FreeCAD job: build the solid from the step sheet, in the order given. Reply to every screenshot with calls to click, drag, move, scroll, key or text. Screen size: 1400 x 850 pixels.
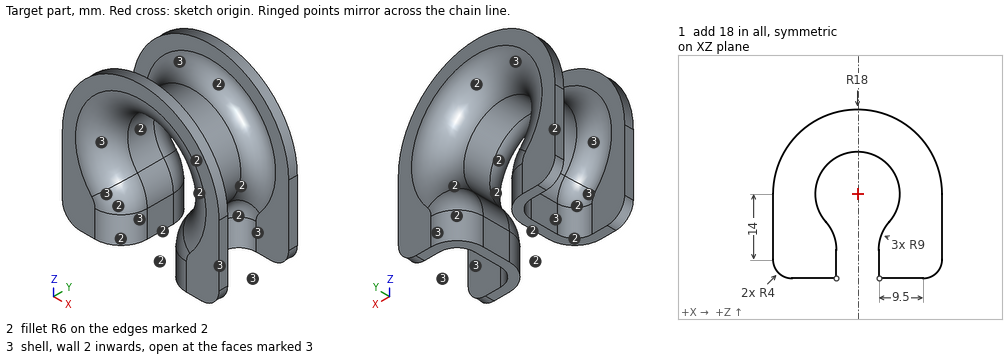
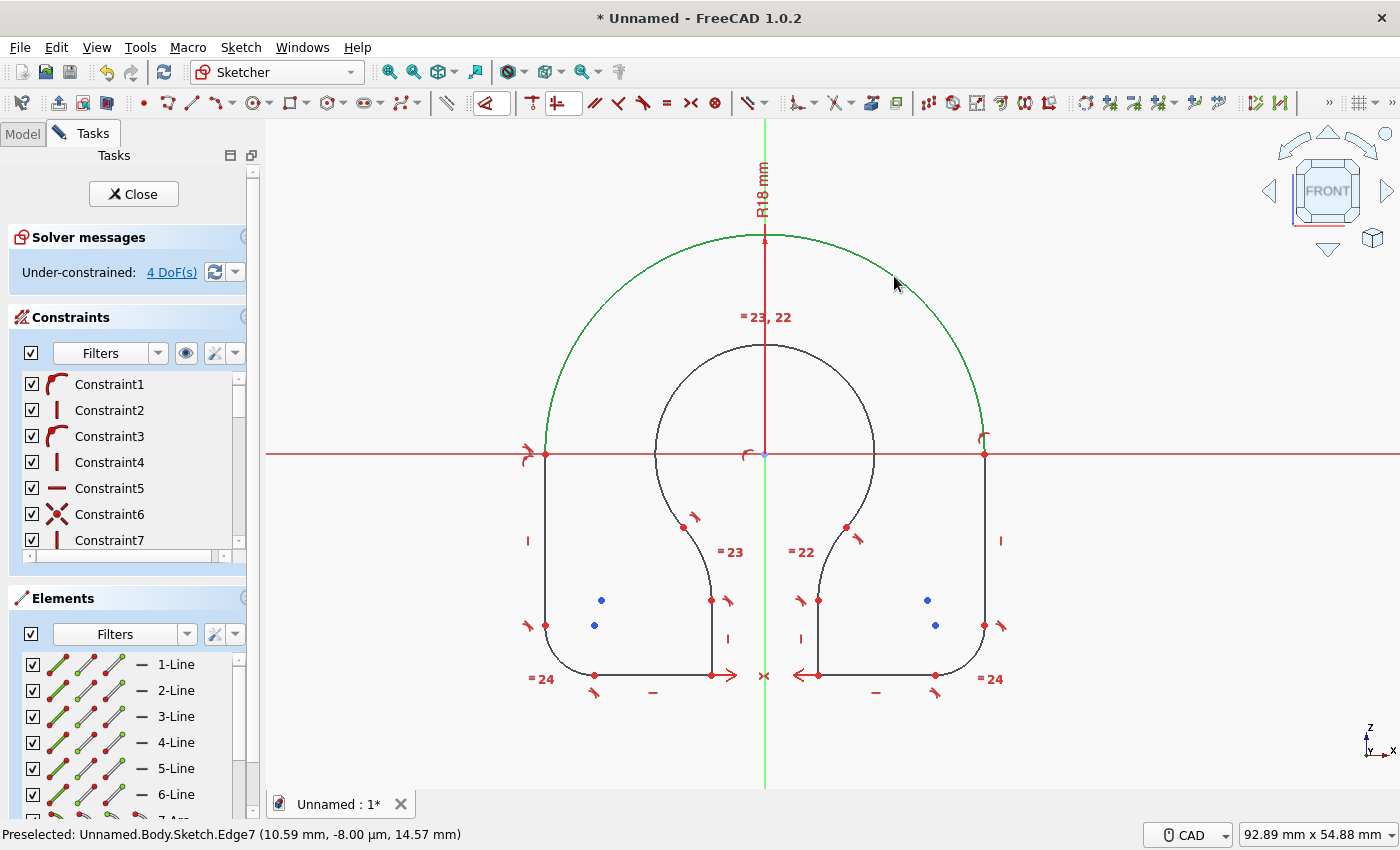
click(958, 670)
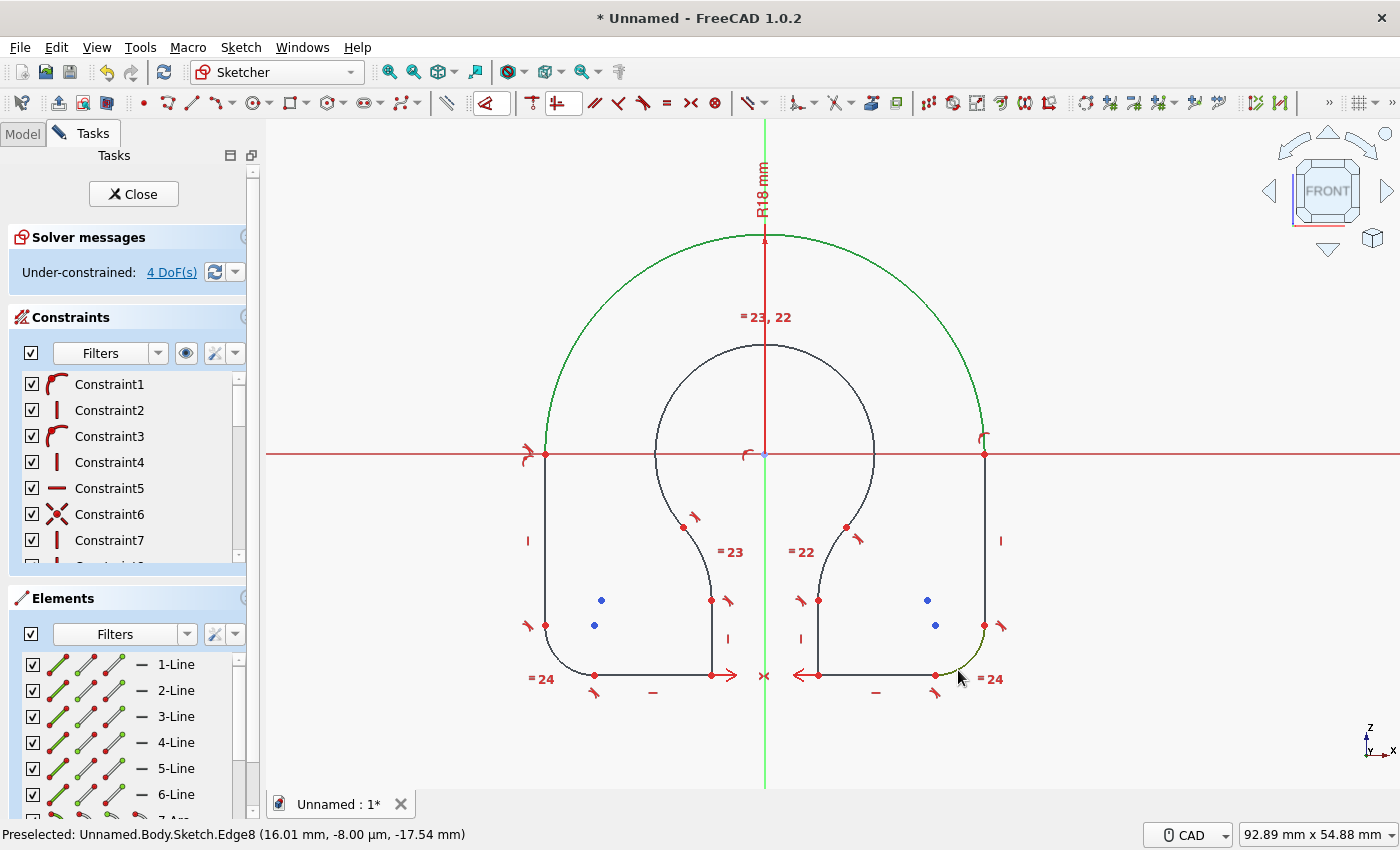
key(k)
key(r)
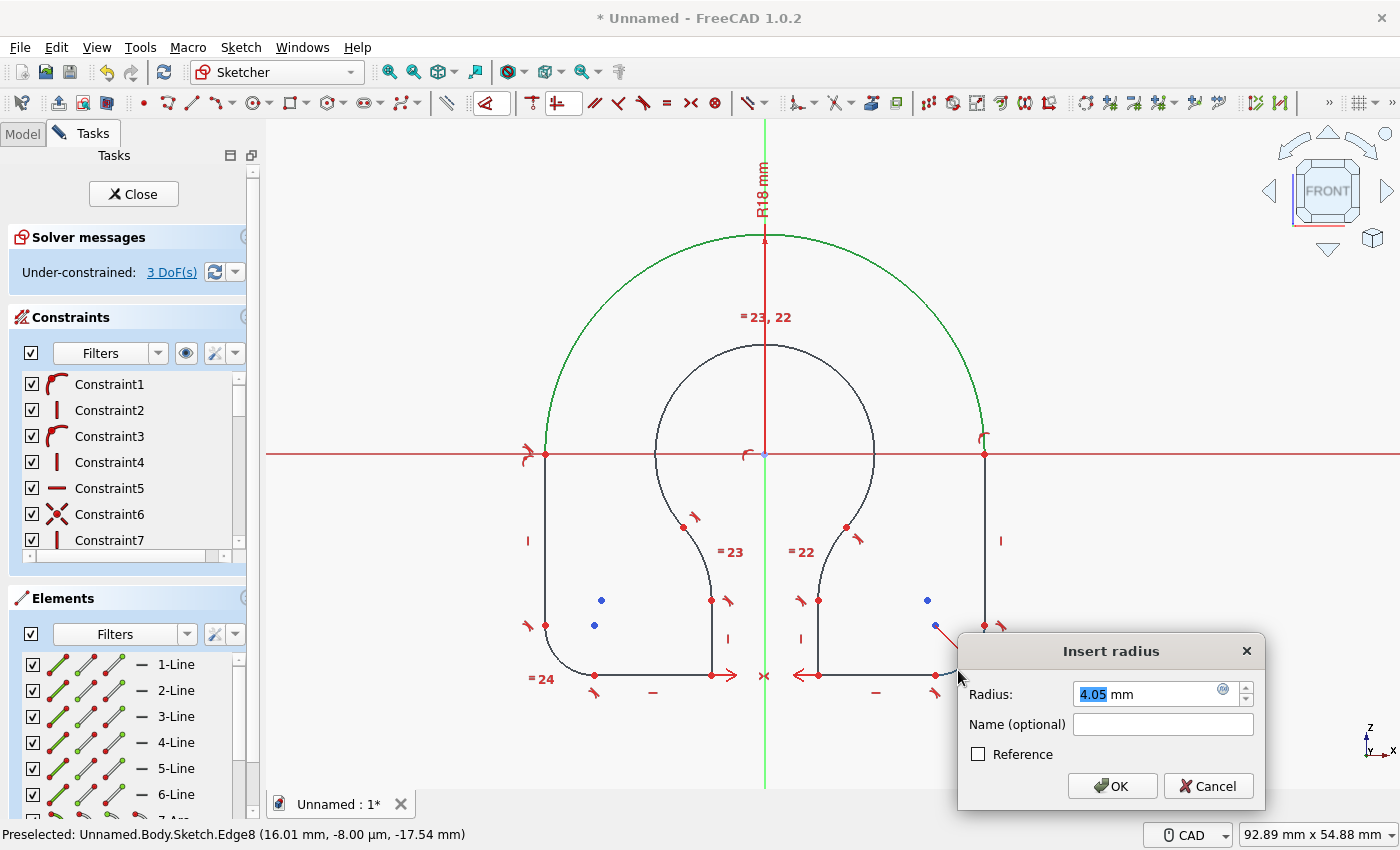
text(4)
key(Return)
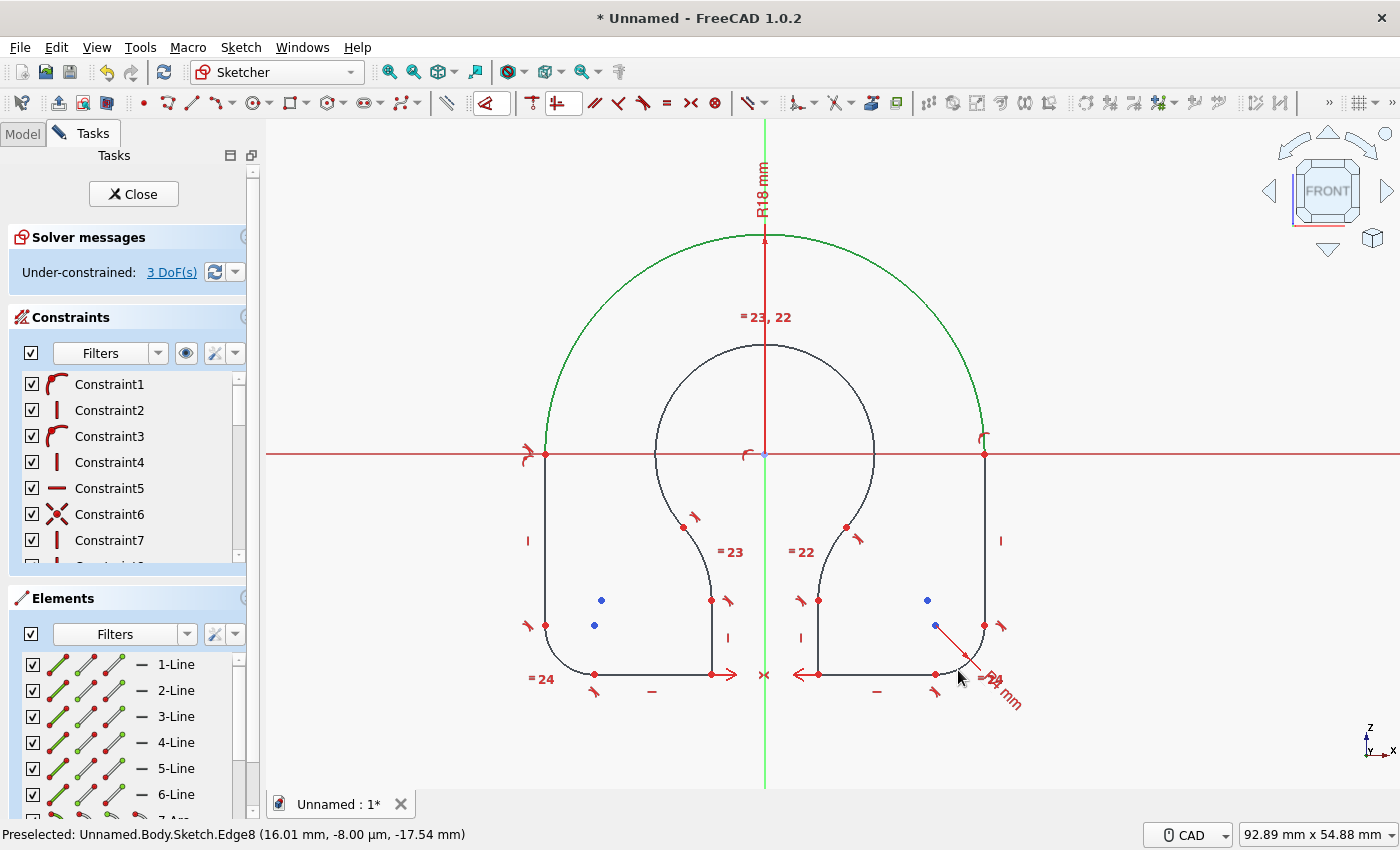
click(832, 547)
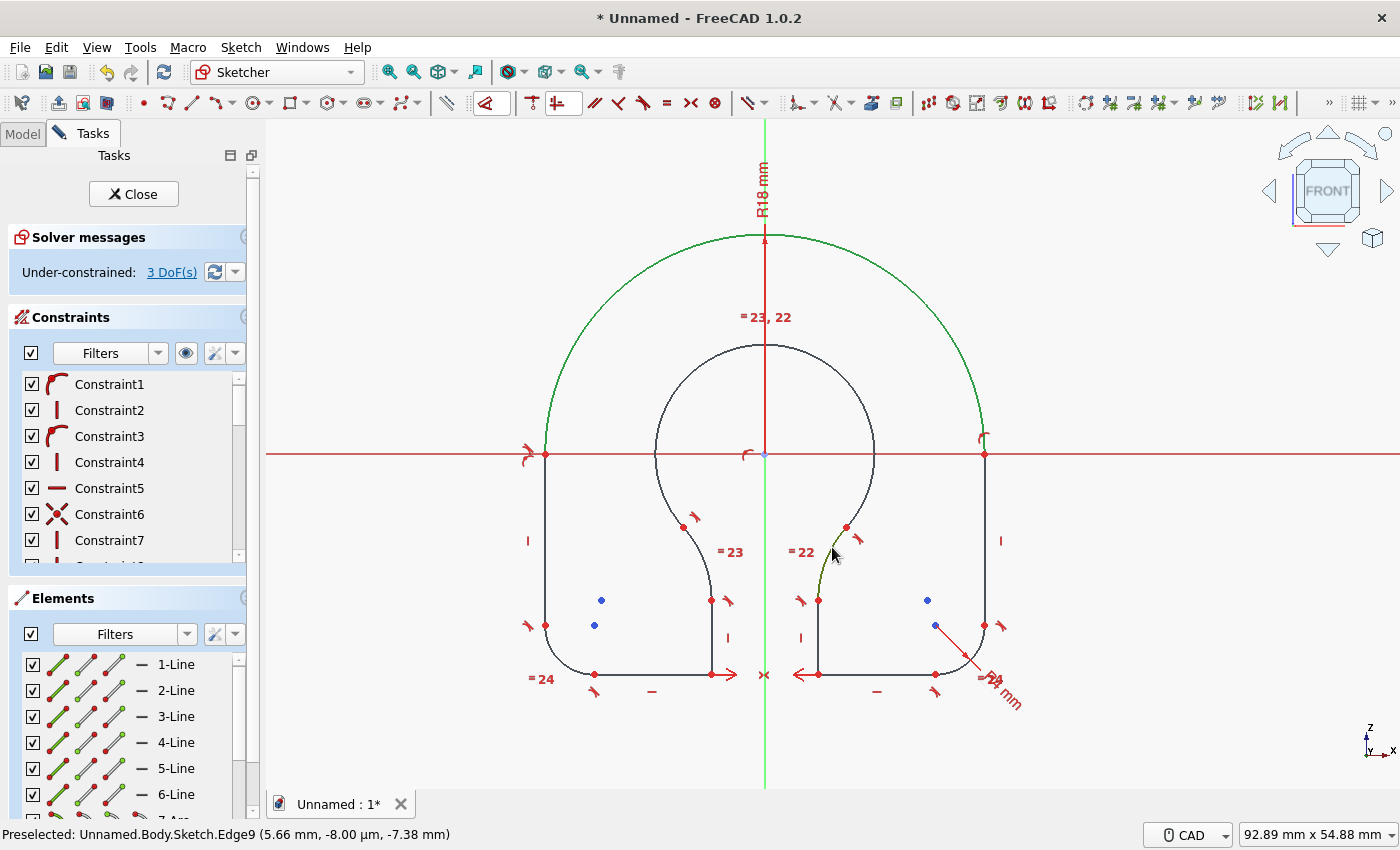
key(k)
key(r)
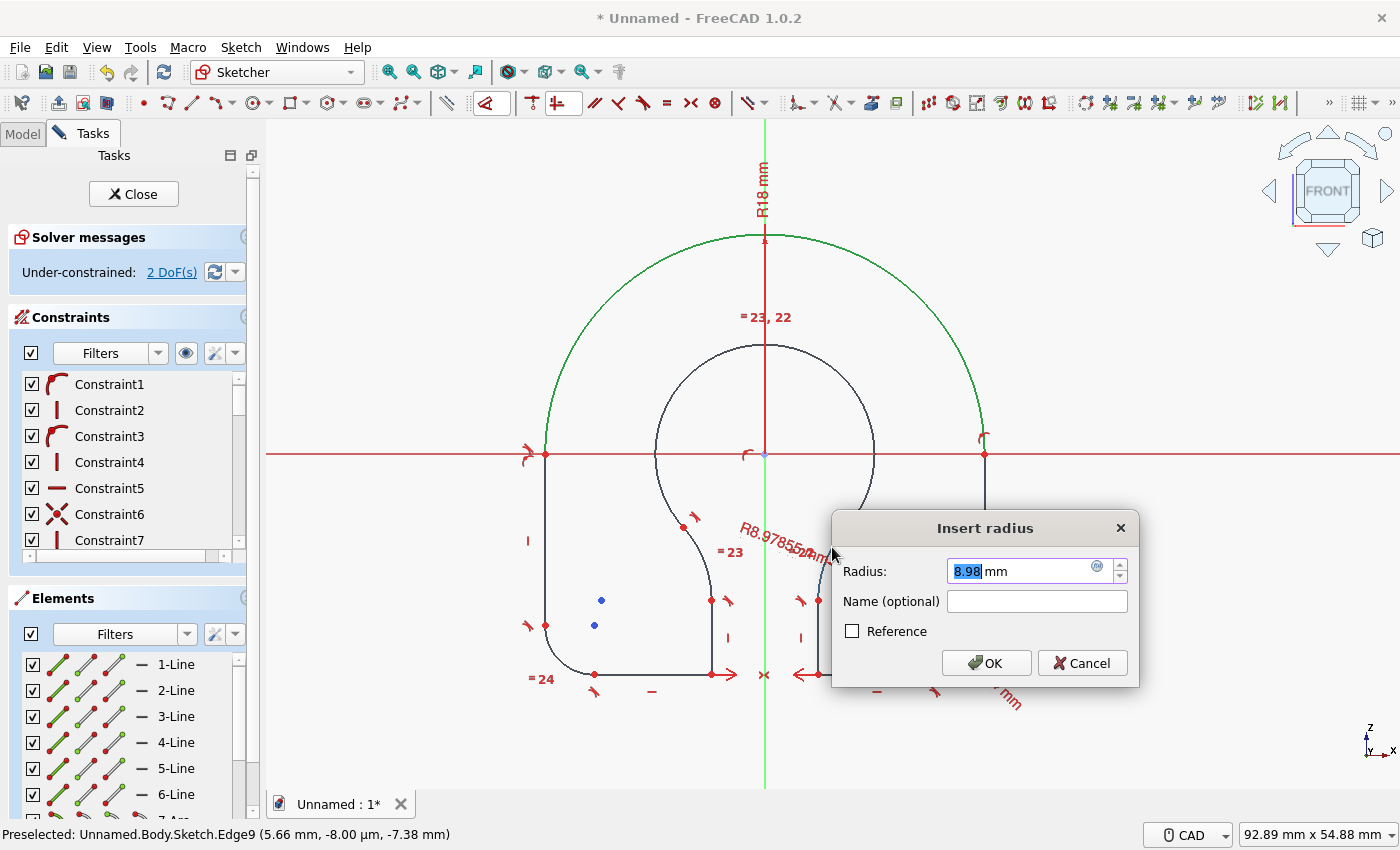
text(9)
key(Return)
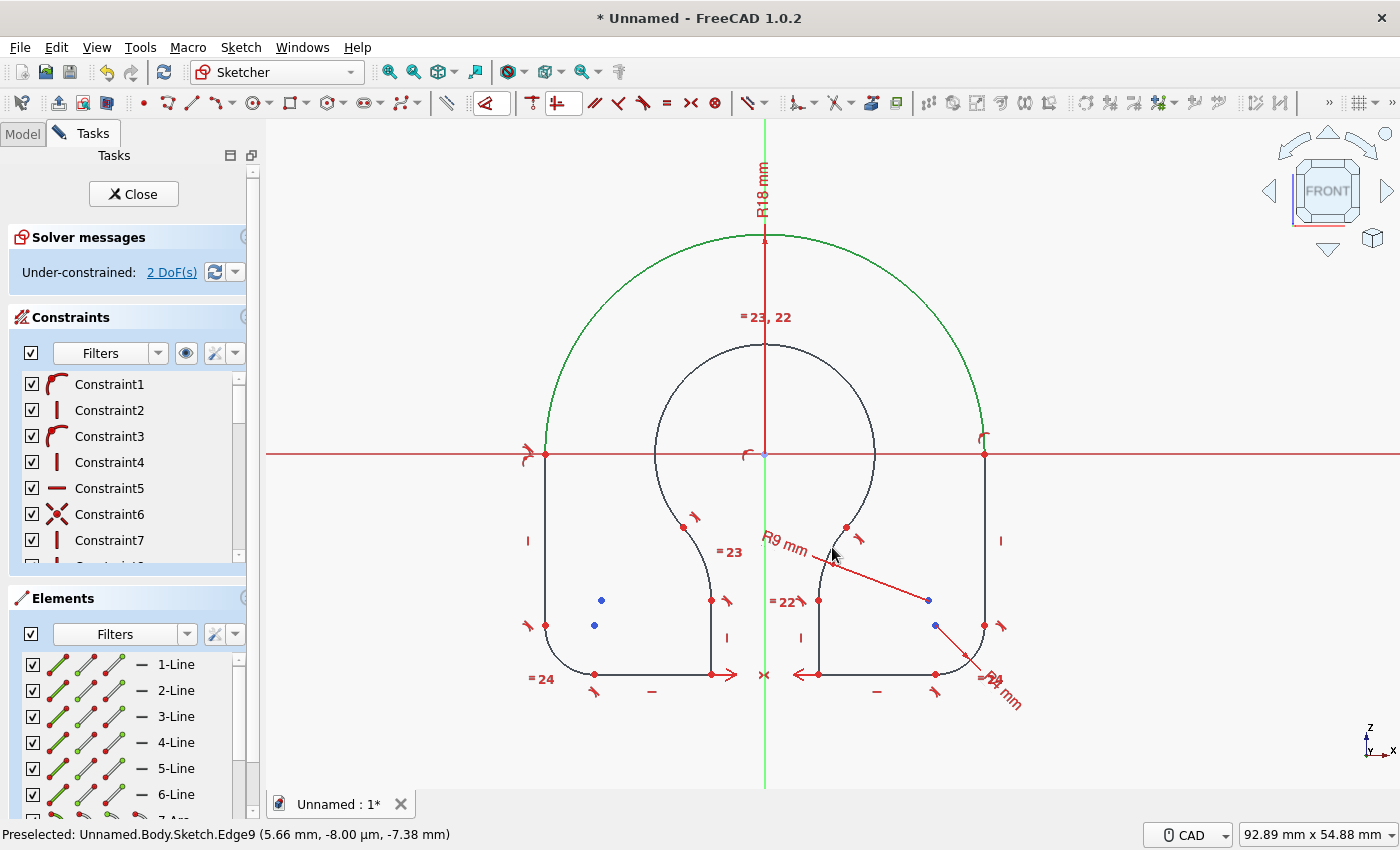
click(545, 574)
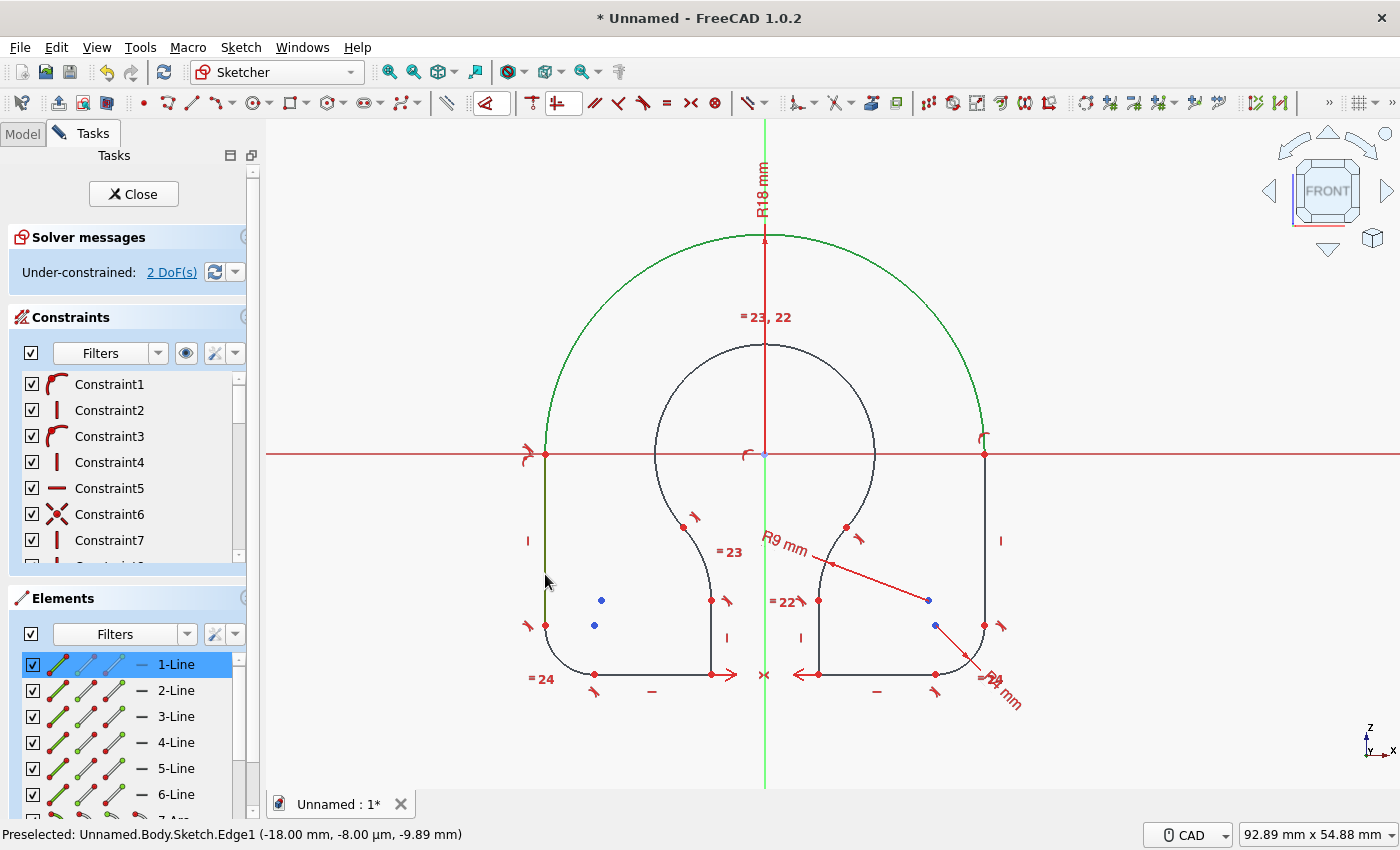
key(i)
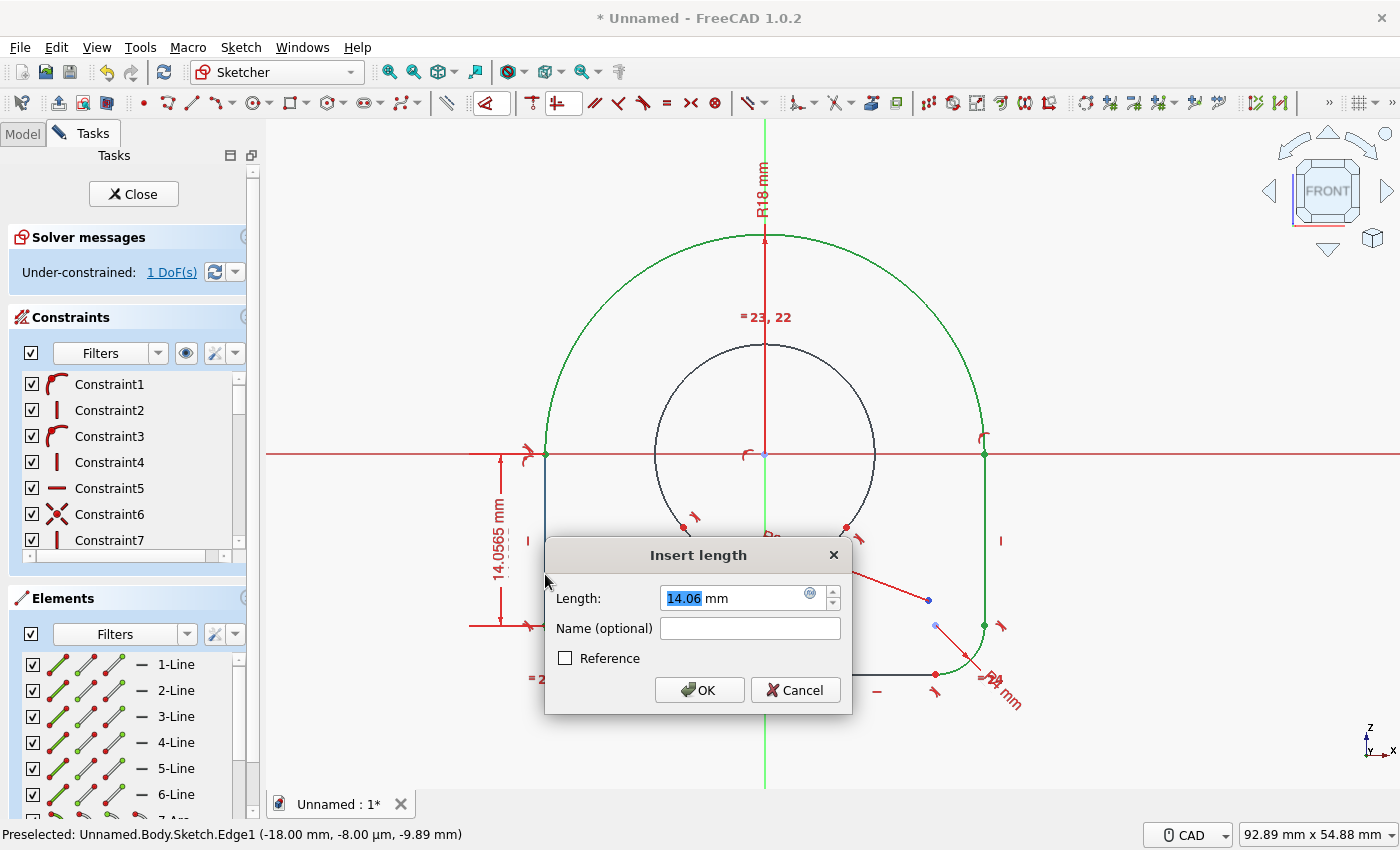
text(14)
key(Return)